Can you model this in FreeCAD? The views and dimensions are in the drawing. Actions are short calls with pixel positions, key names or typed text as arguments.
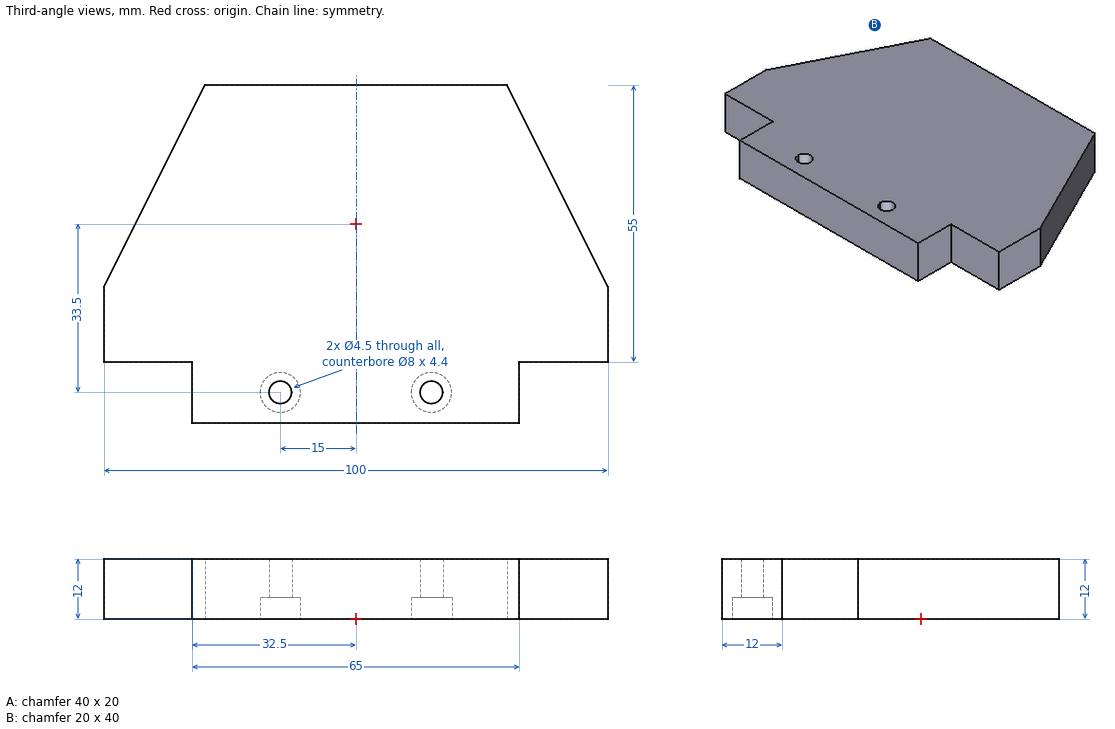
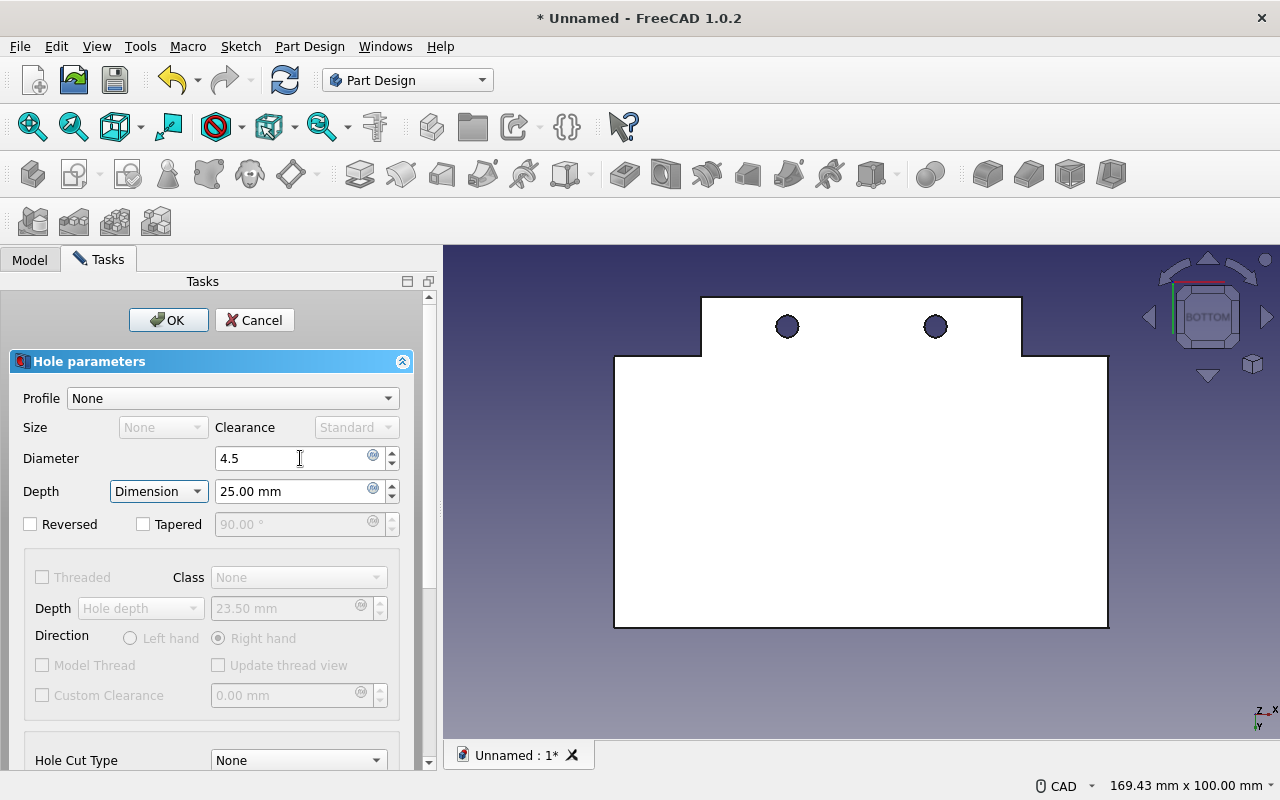
click(160, 492)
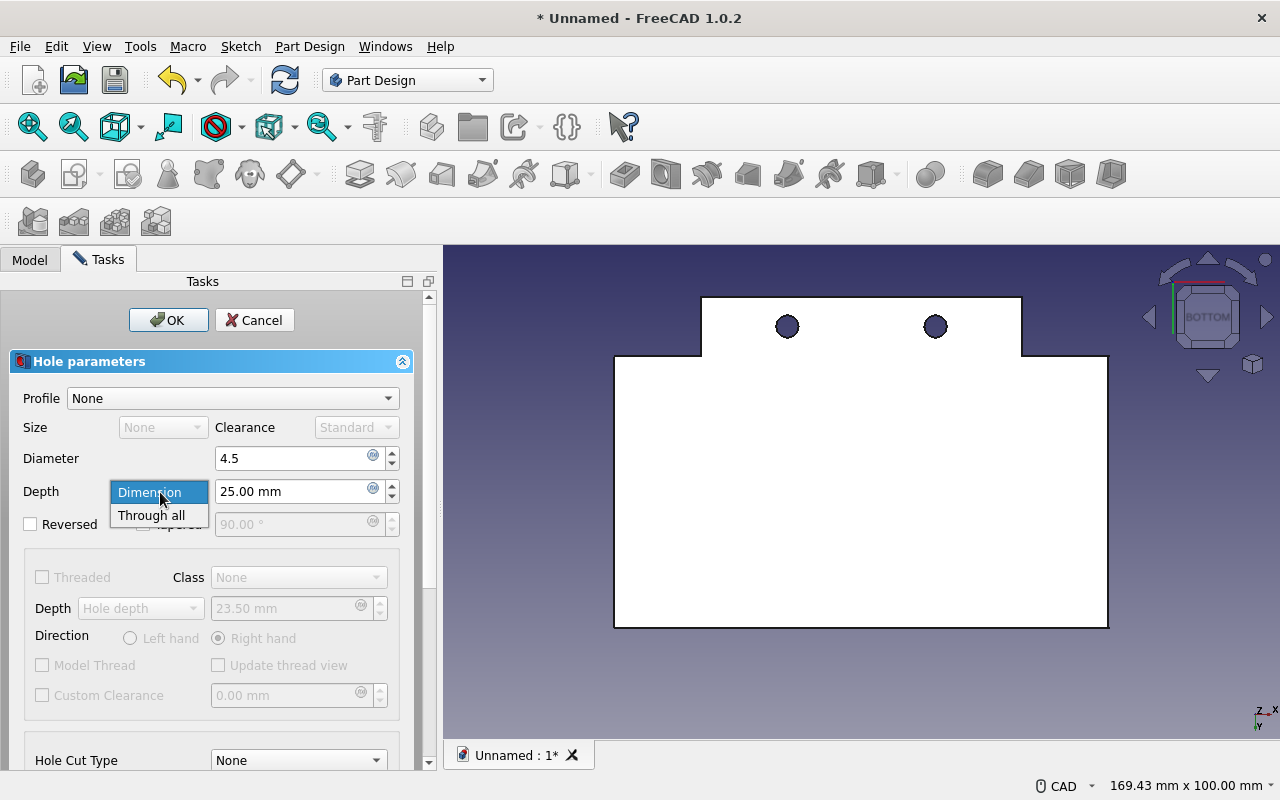
click(158, 516)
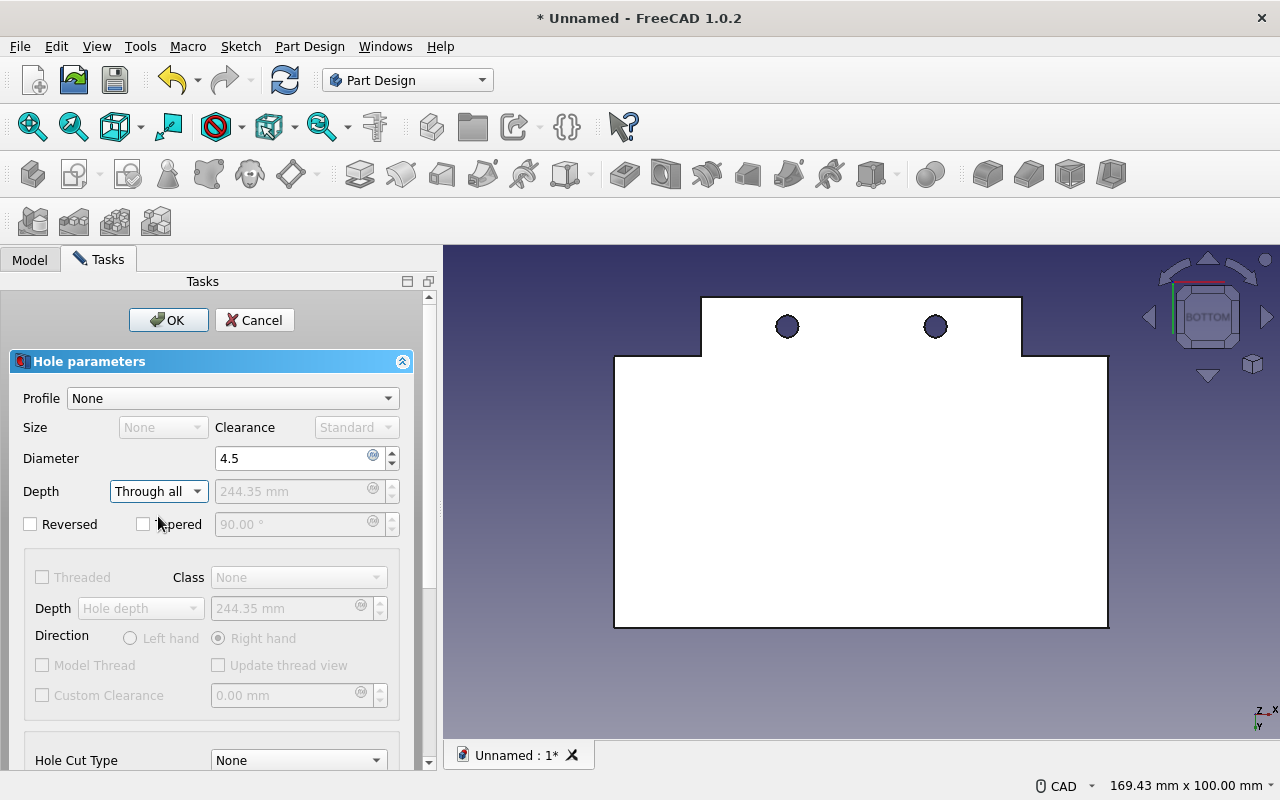
scroll(429, 530, down, 2)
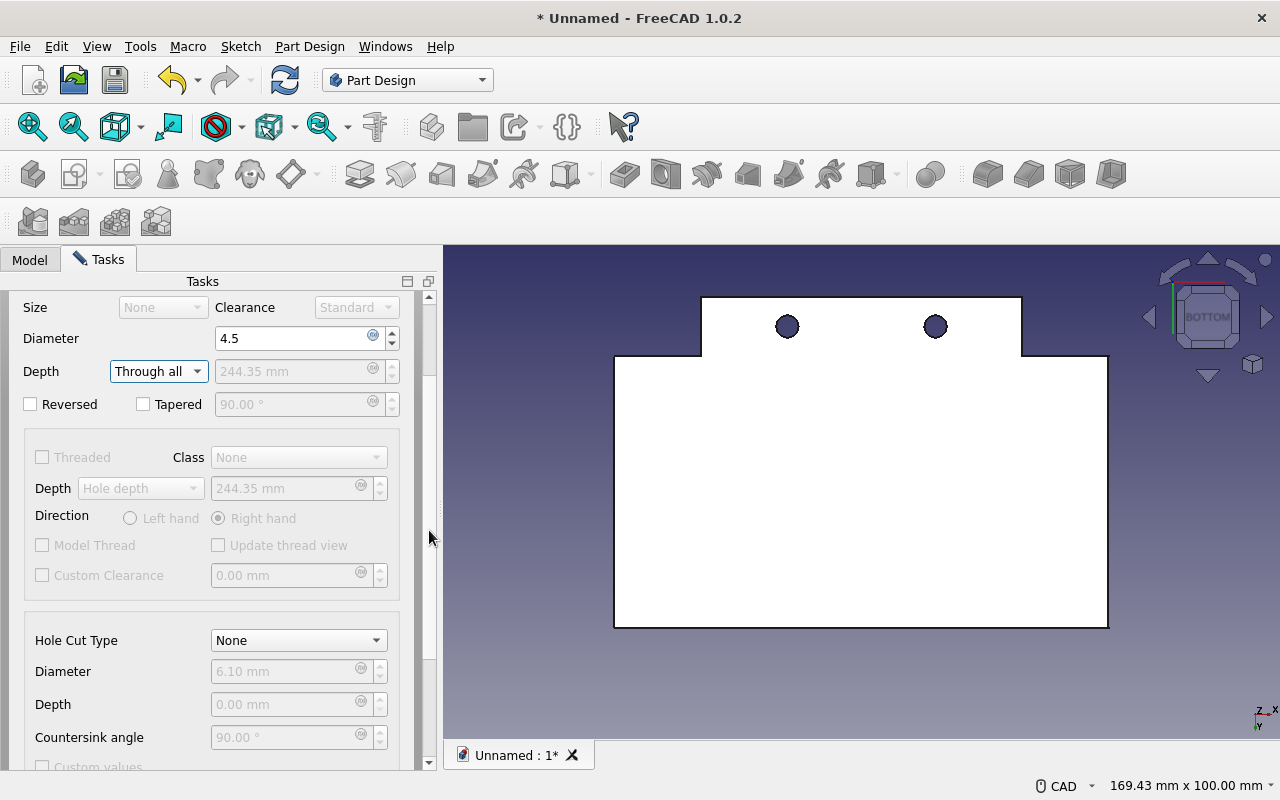
click(300, 640)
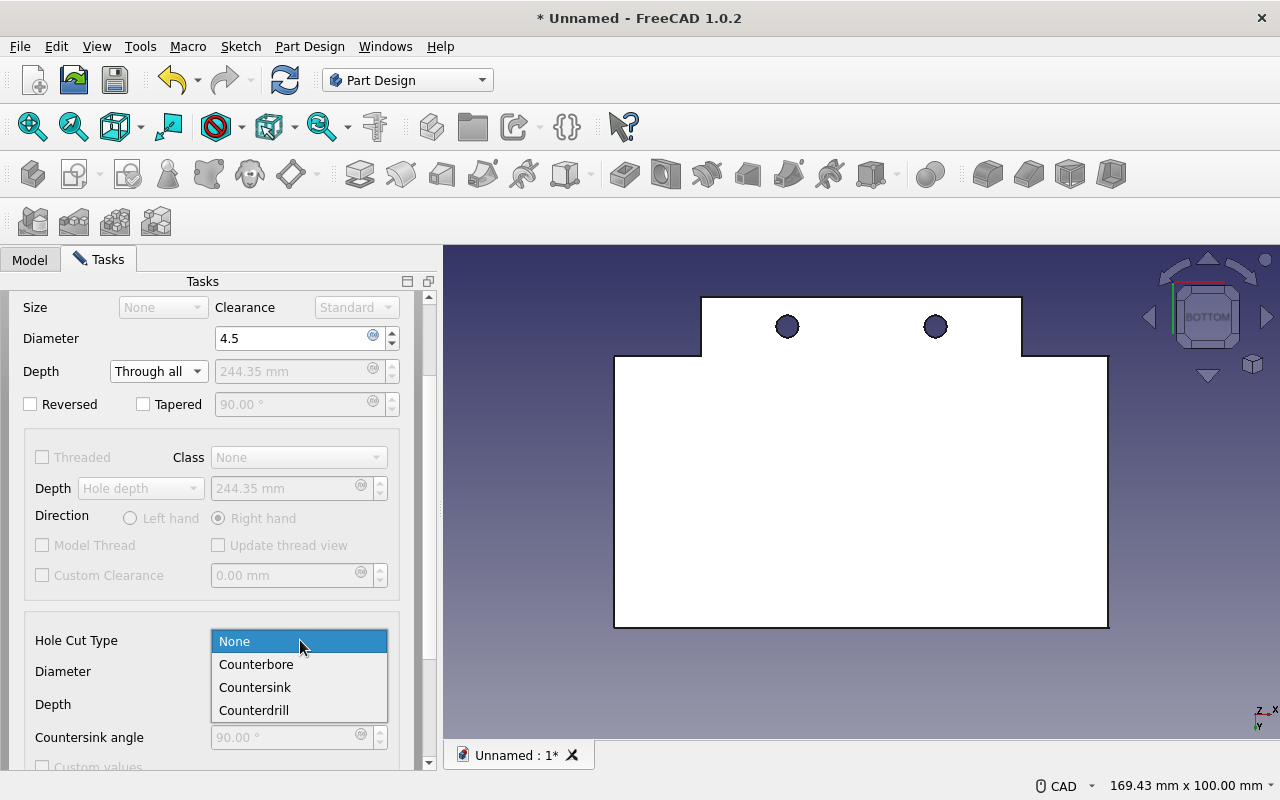
click(298, 664)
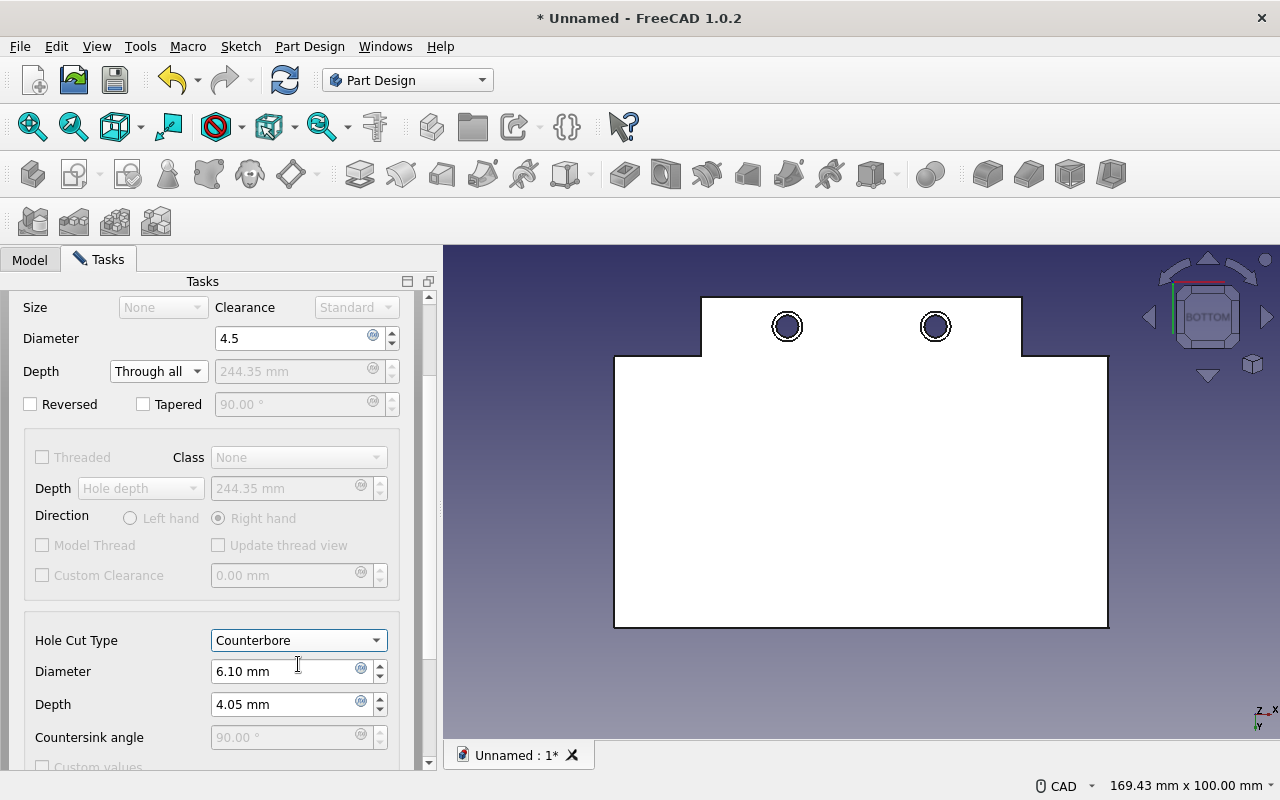
triple_click(292, 672)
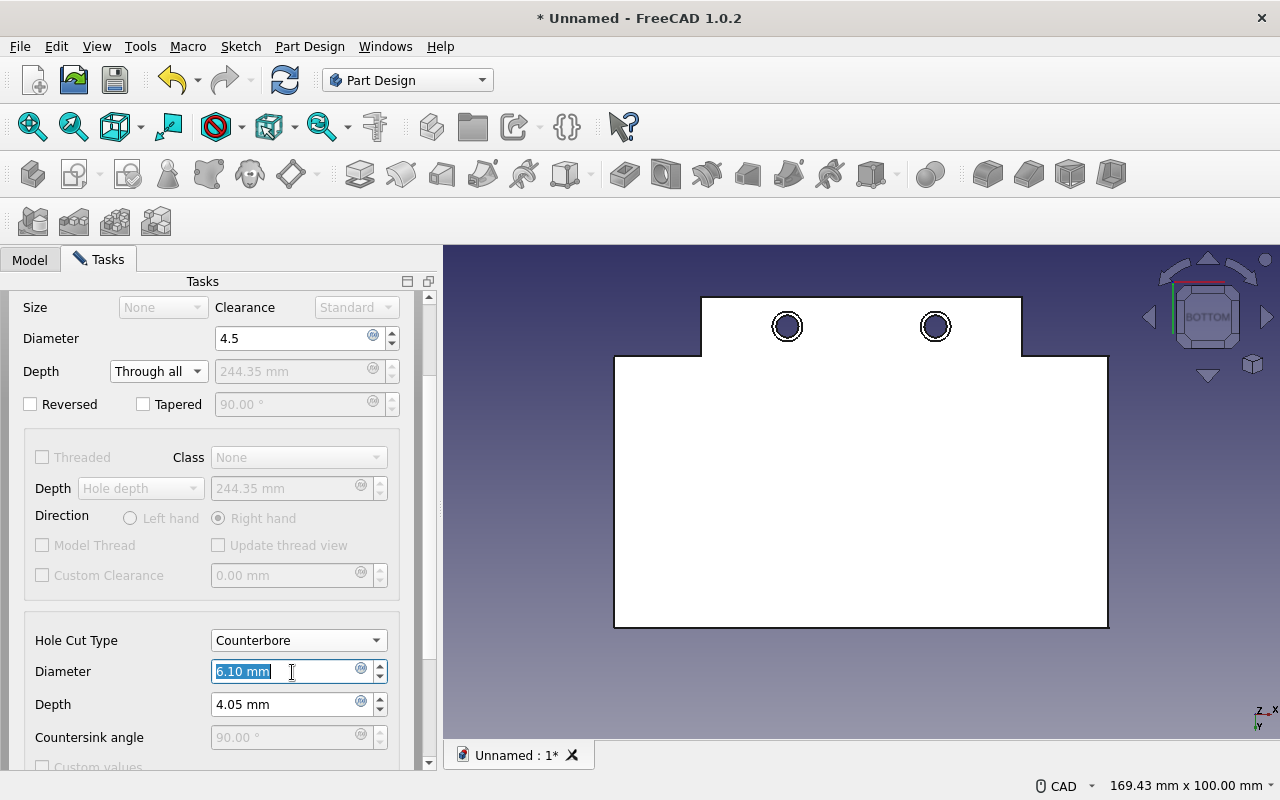
text(8)
key(Tab)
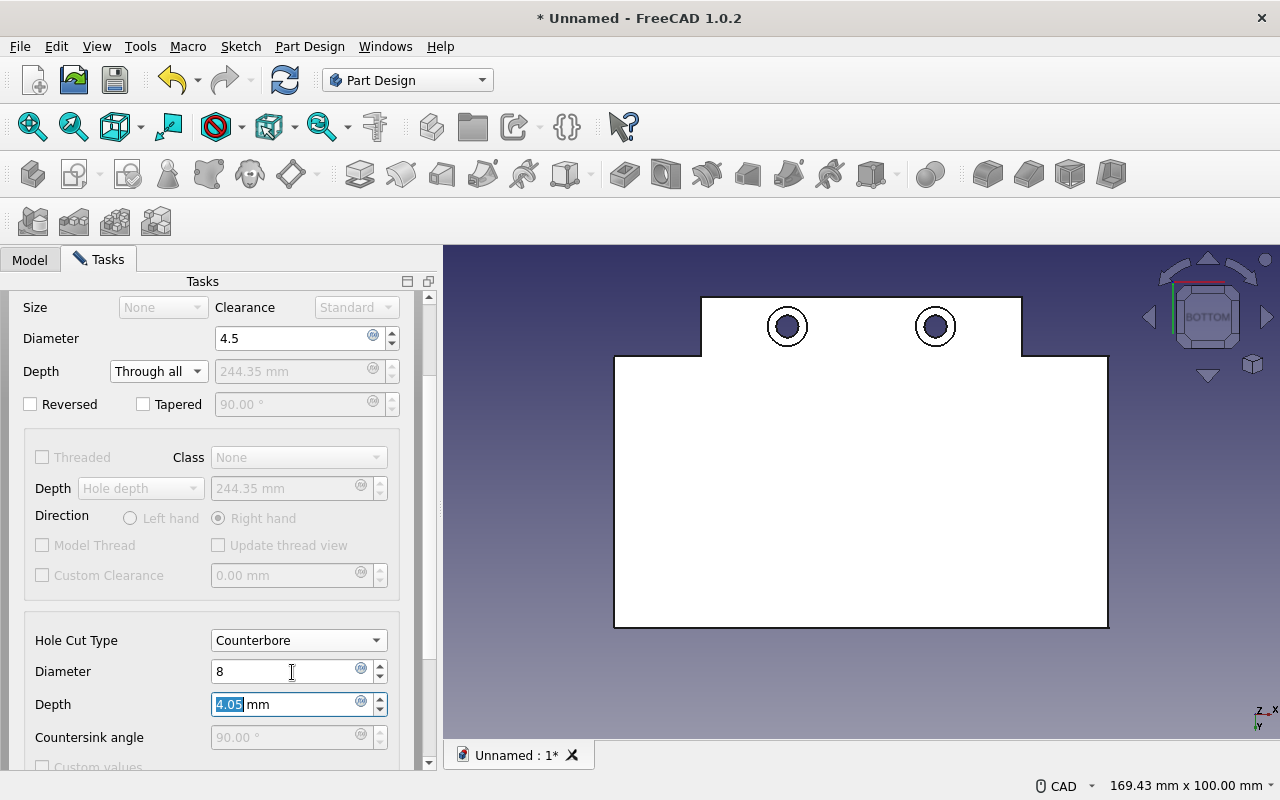
text(4.4)
key(Tab)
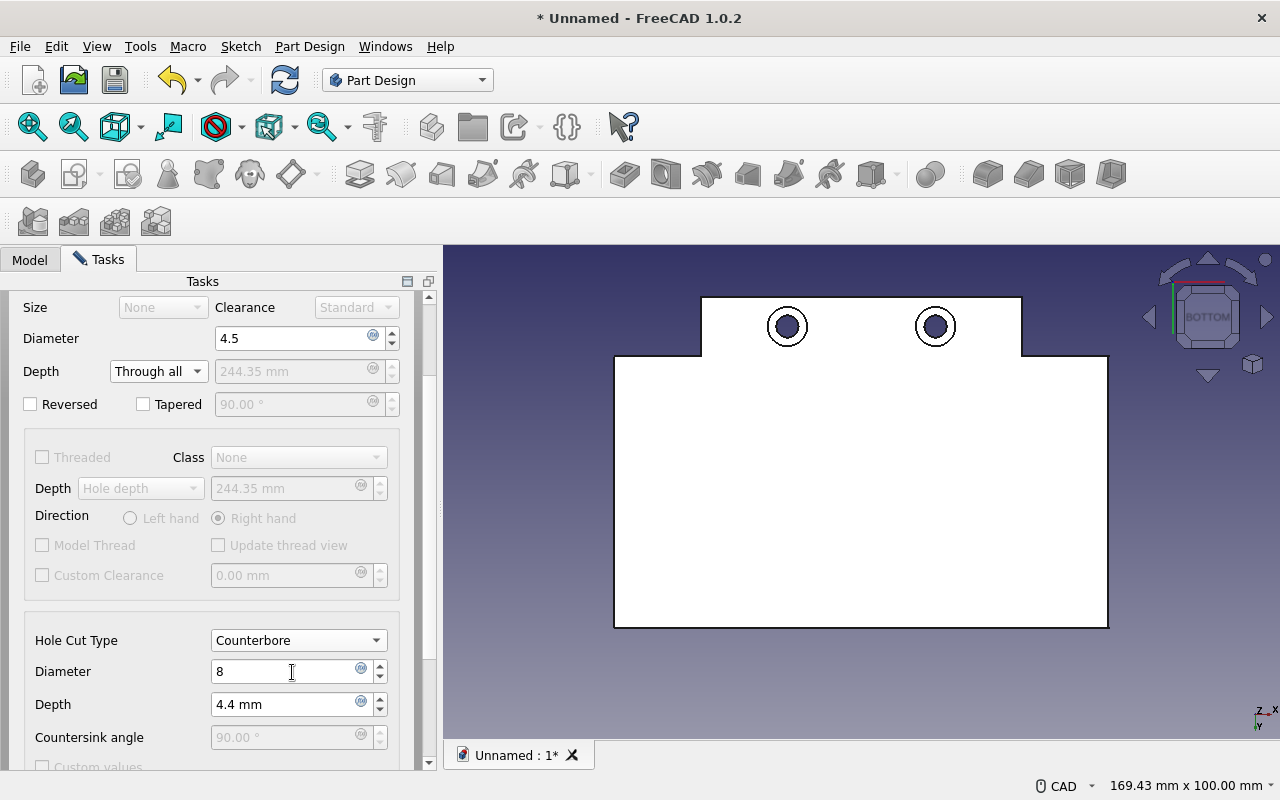
scroll(429, 530, up, 3)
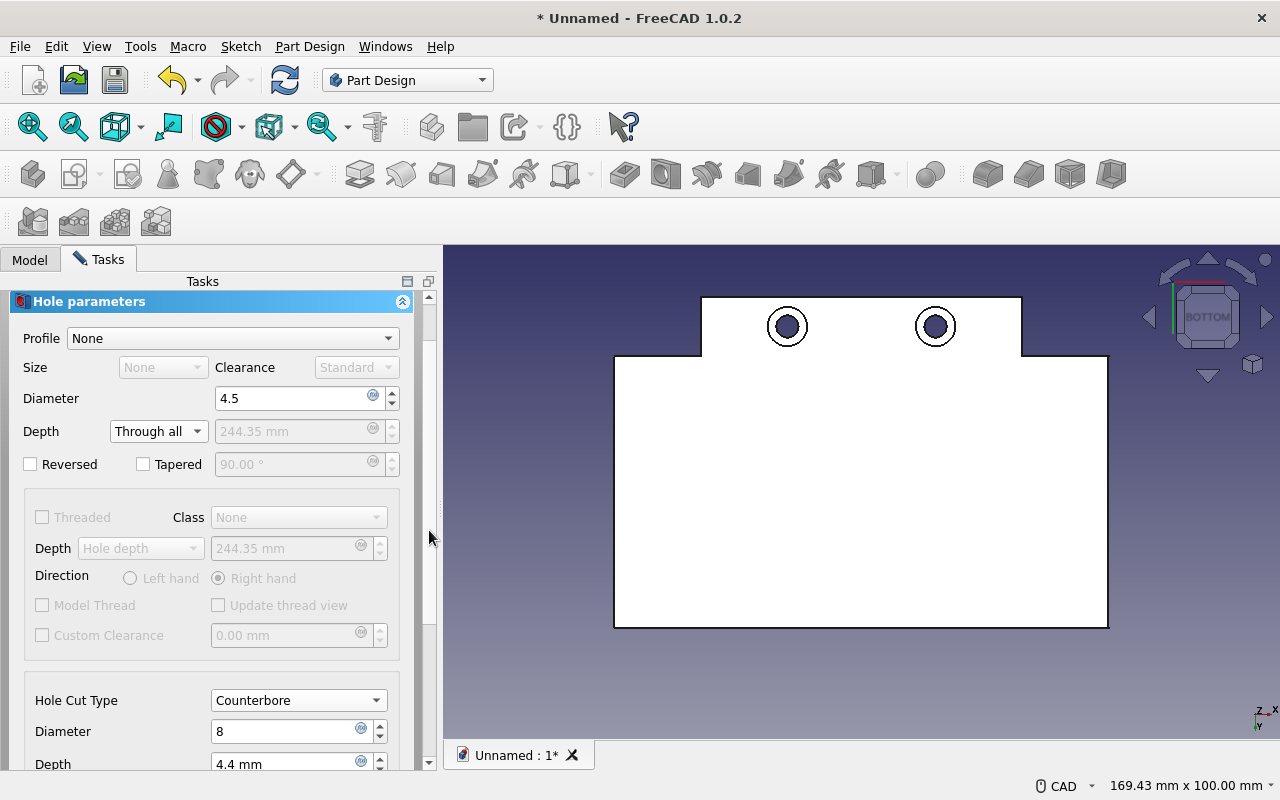
click(169, 320)